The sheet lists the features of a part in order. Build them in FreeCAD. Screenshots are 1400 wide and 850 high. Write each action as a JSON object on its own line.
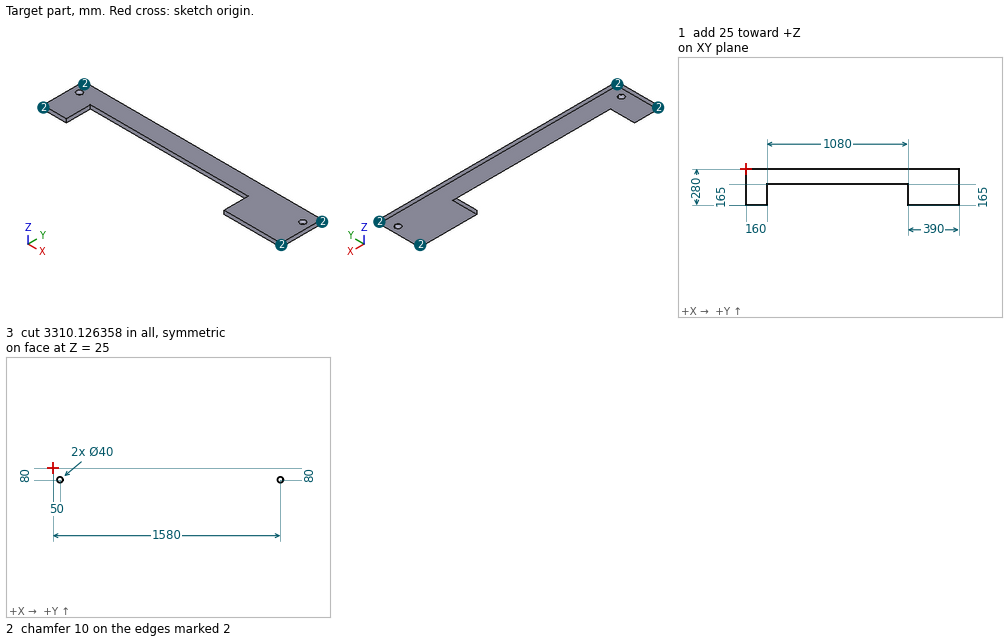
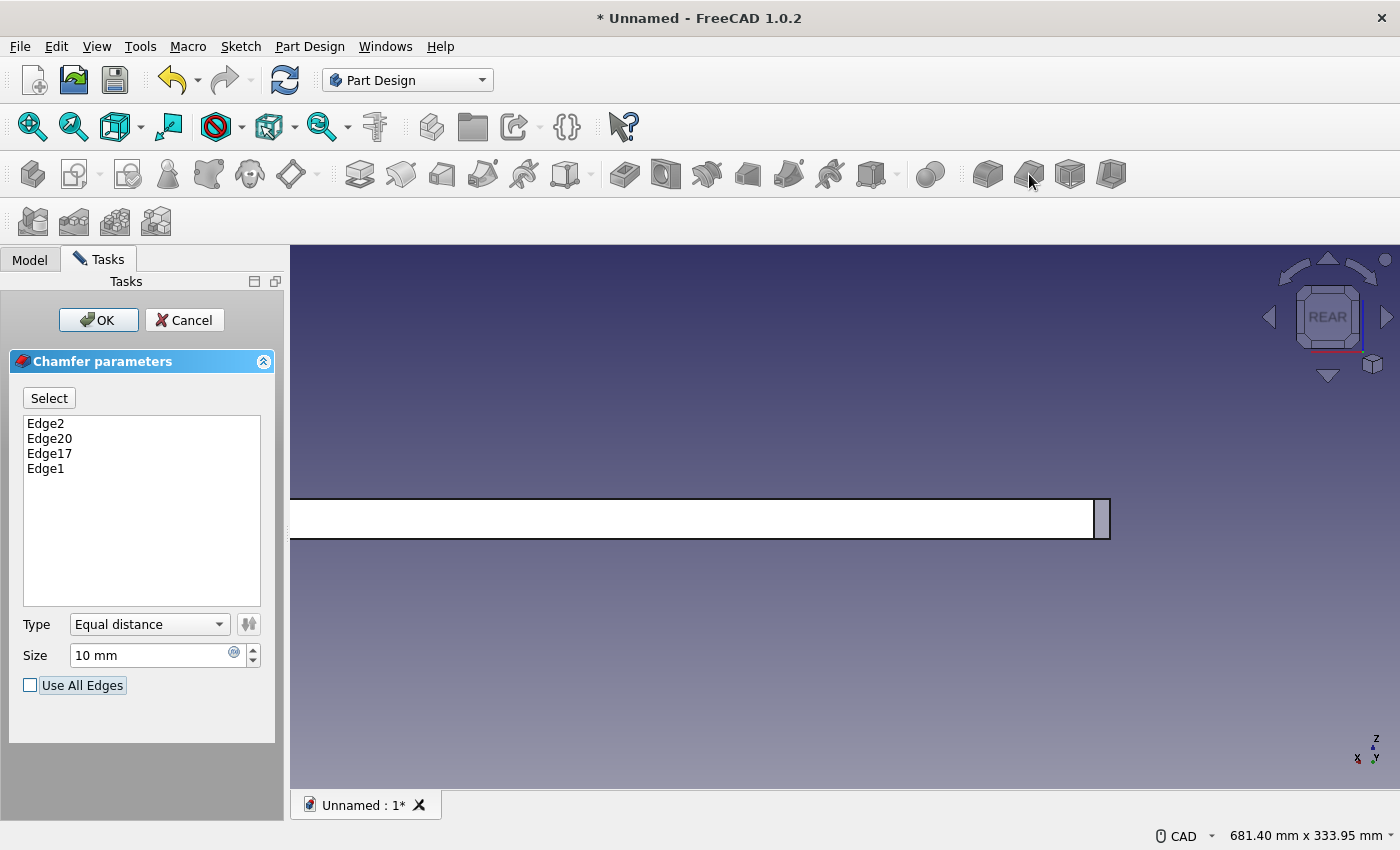
{"action": "left_click", "coordinate": [99, 320]}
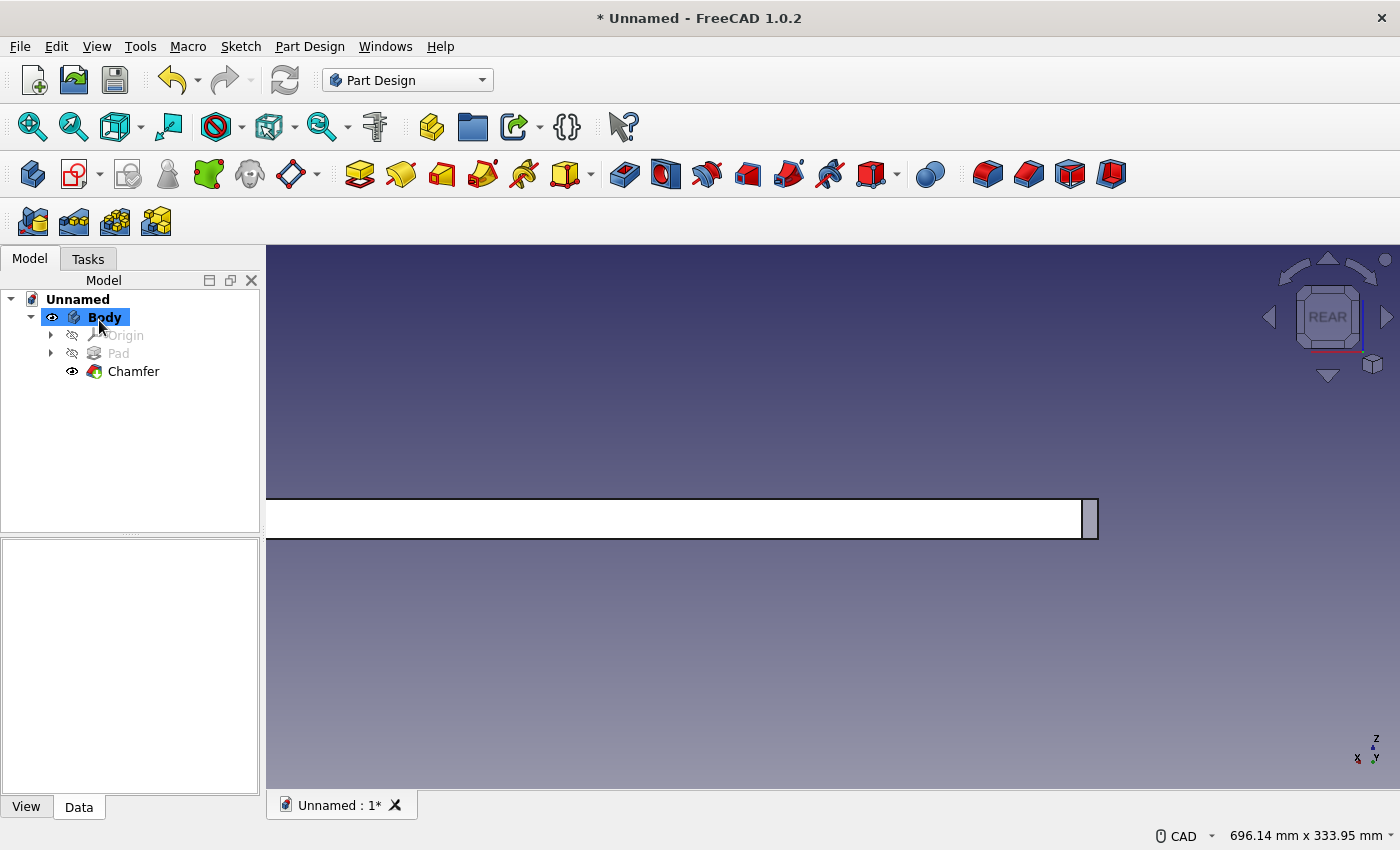
{"action": "key", "text": "v f"}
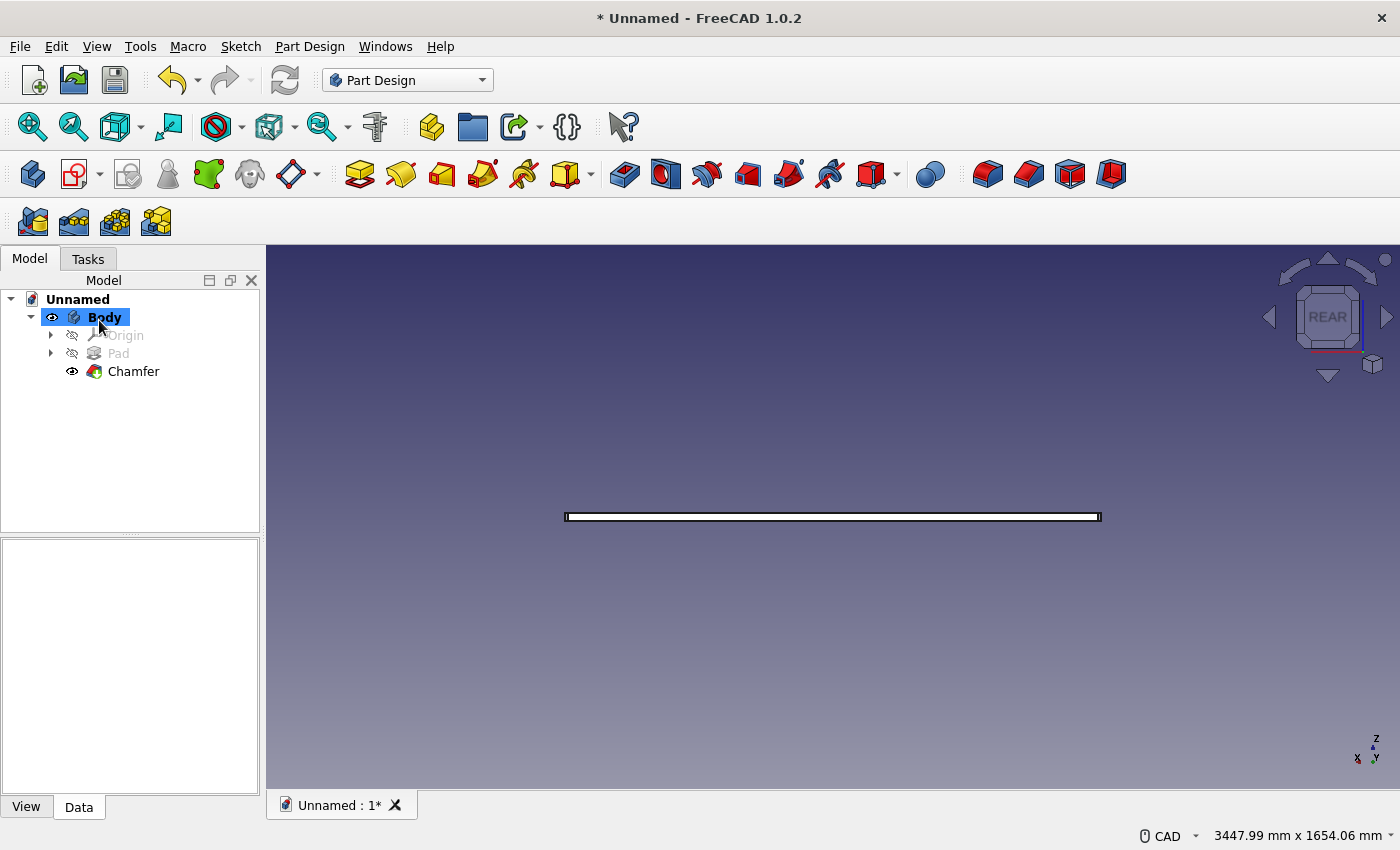
{"action": "key", "text": "0"}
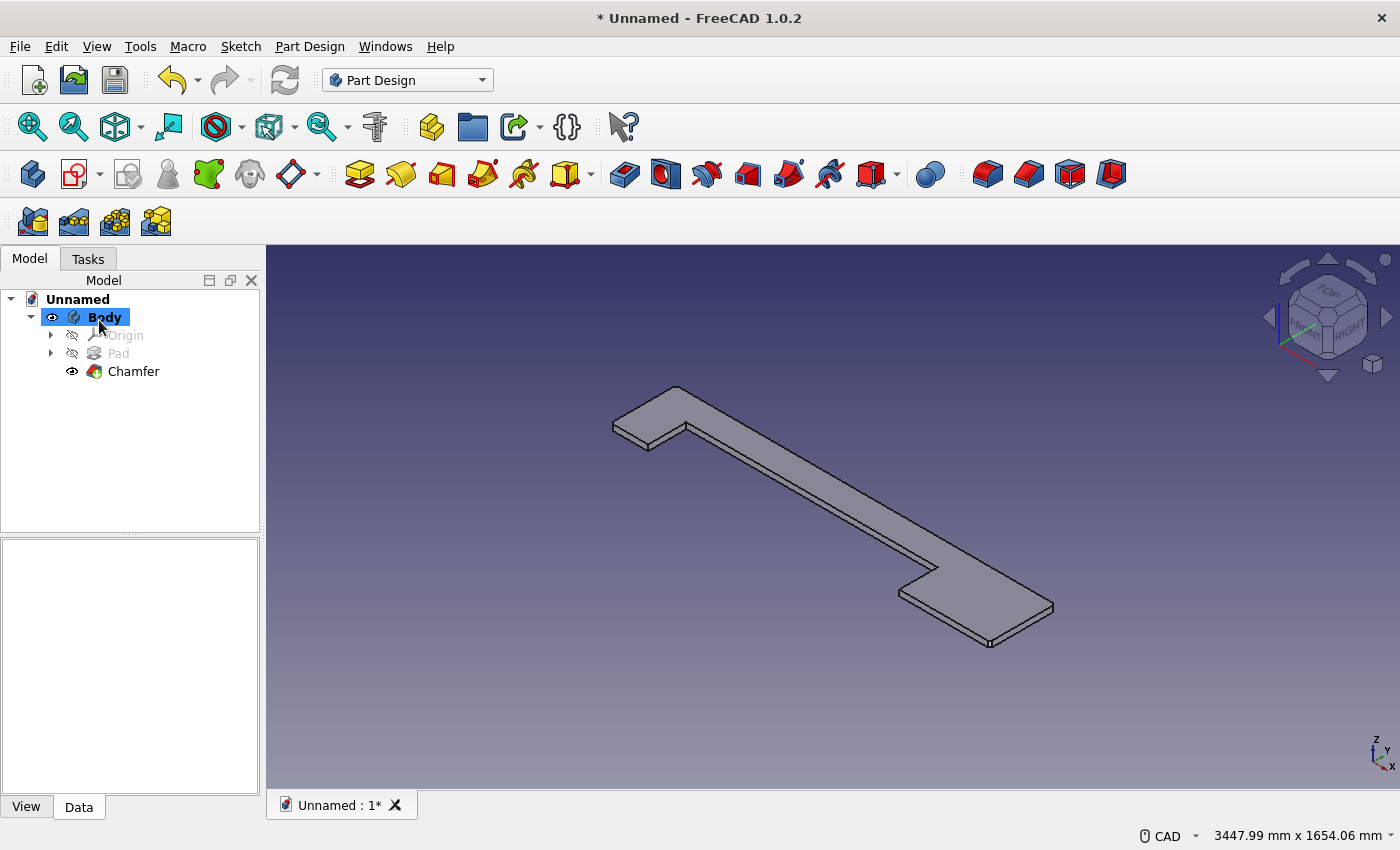
{"action": "left_click", "coordinate": [995, 606]}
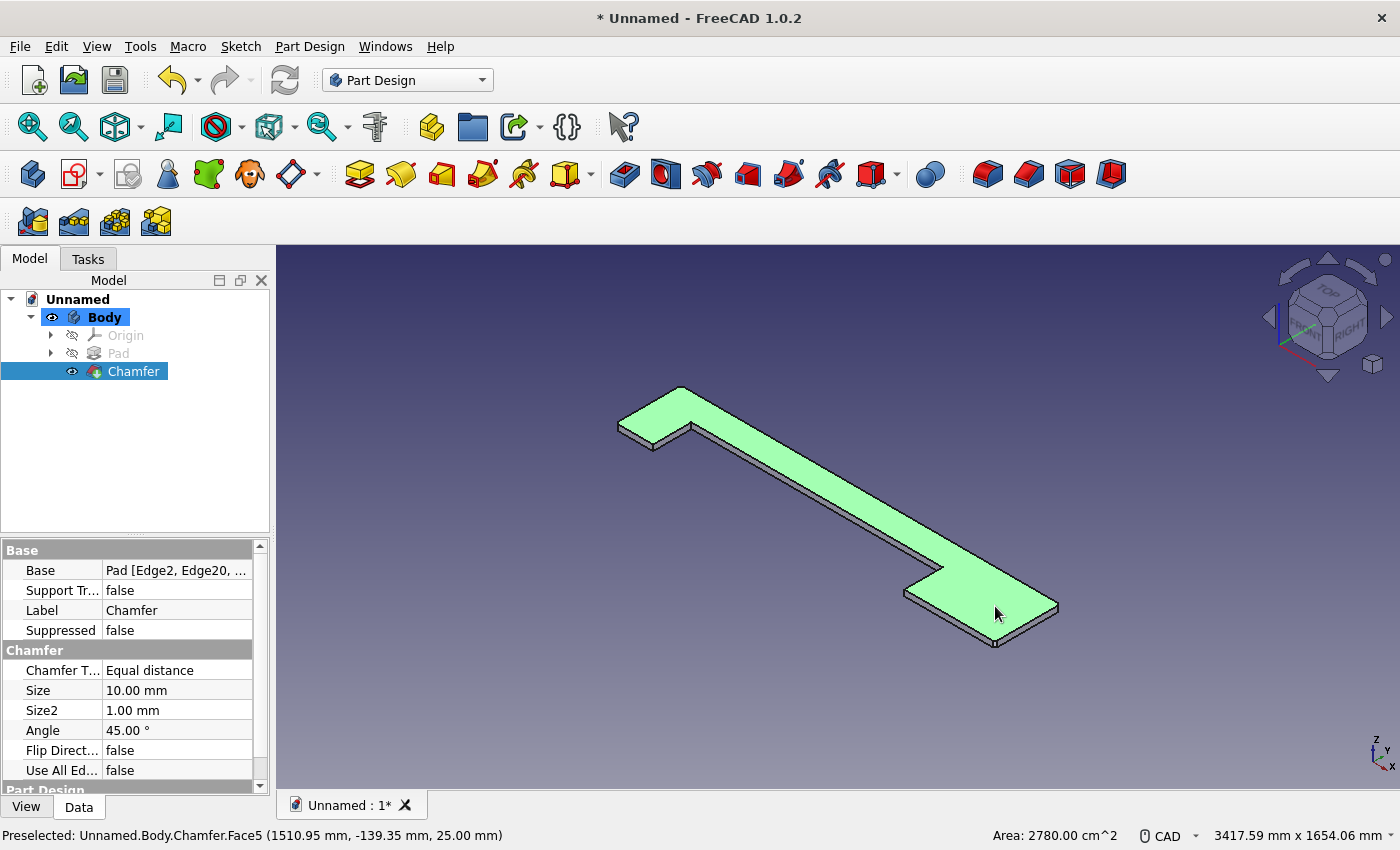
{"action": "left_click", "coordinate": [74, 174]}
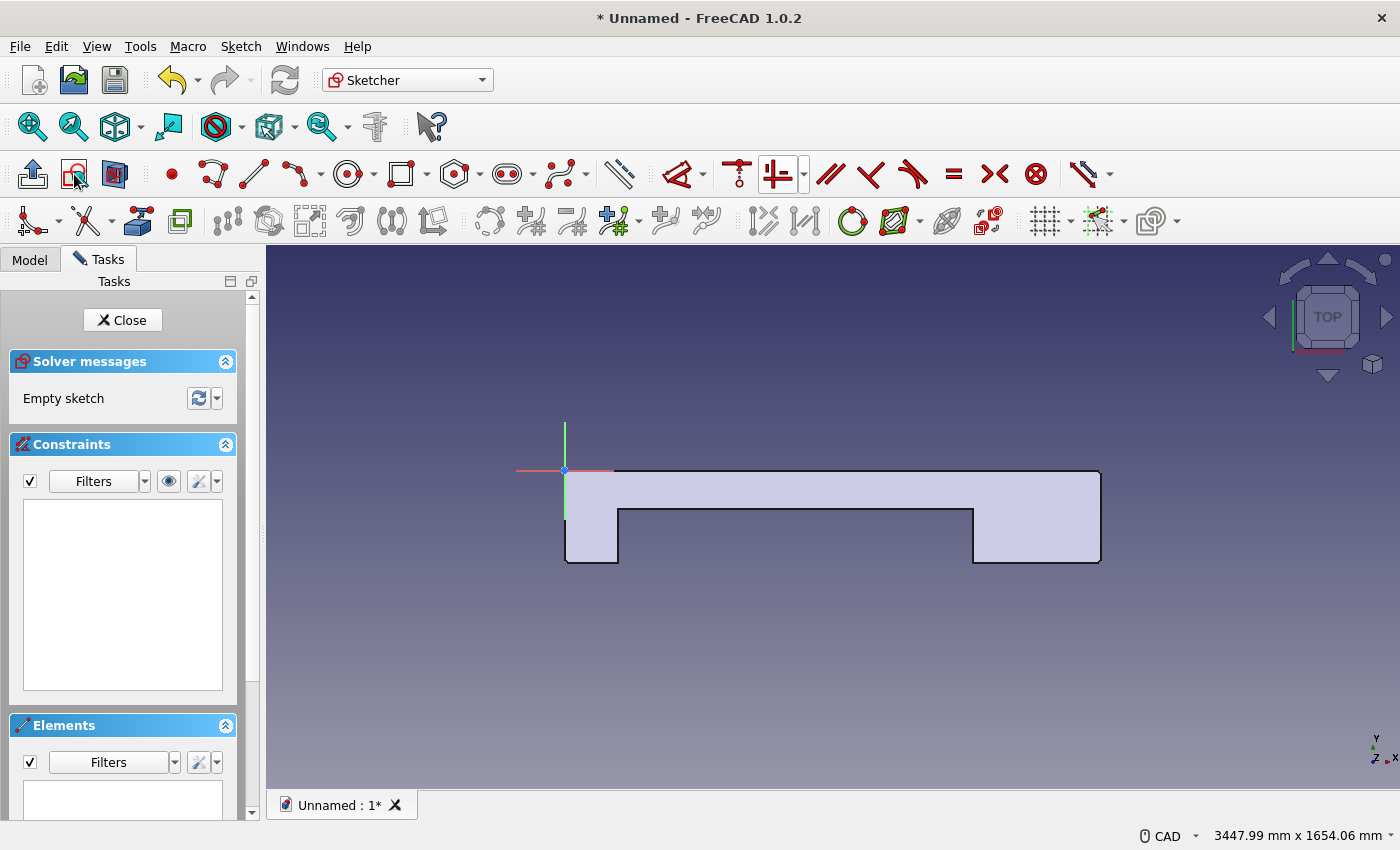
{"action": "key", "text": "g c"}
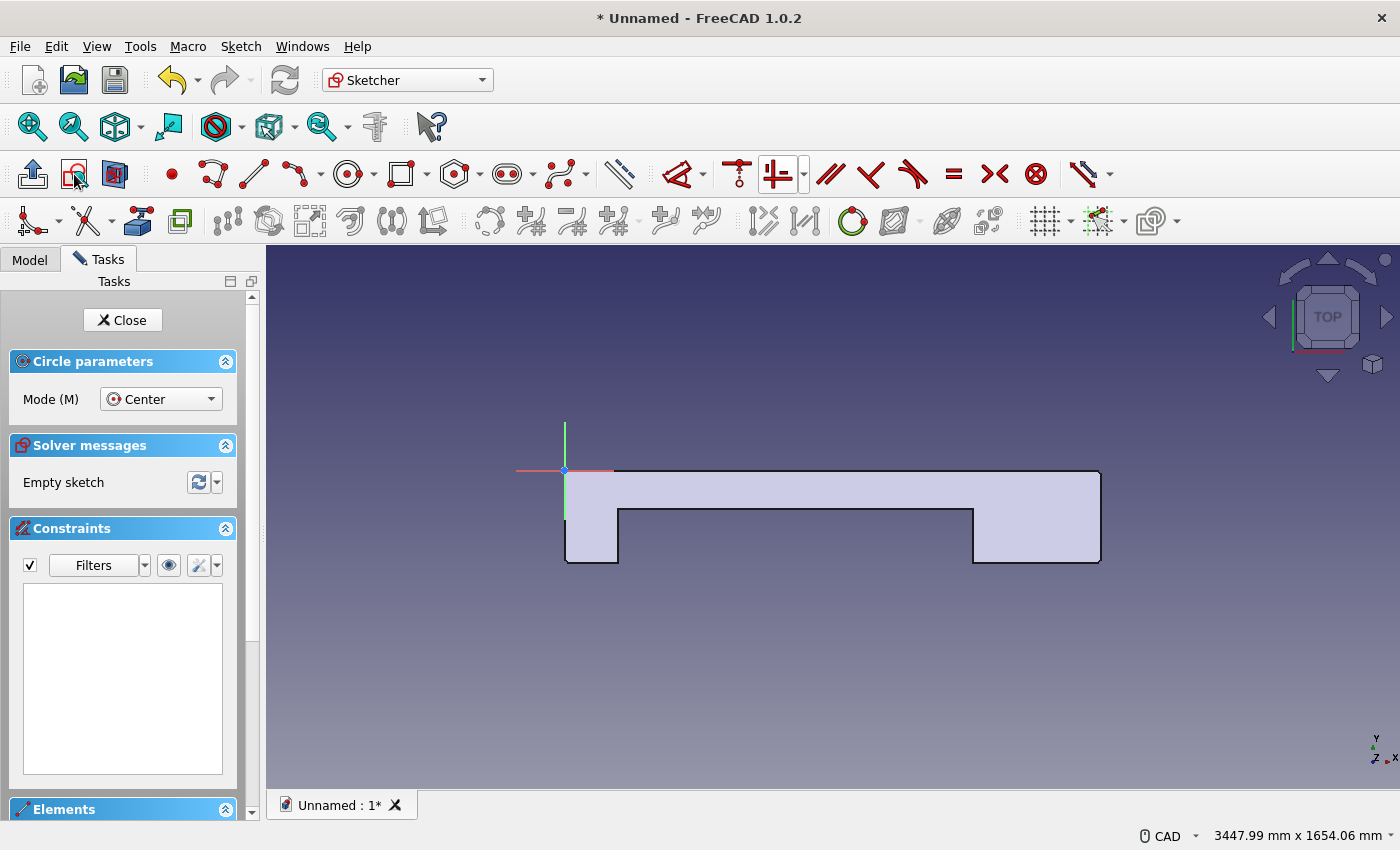
{"action": "scroll", "coordinate": [581, 497], "scroll_direction": "up", "scroll_amount": 7}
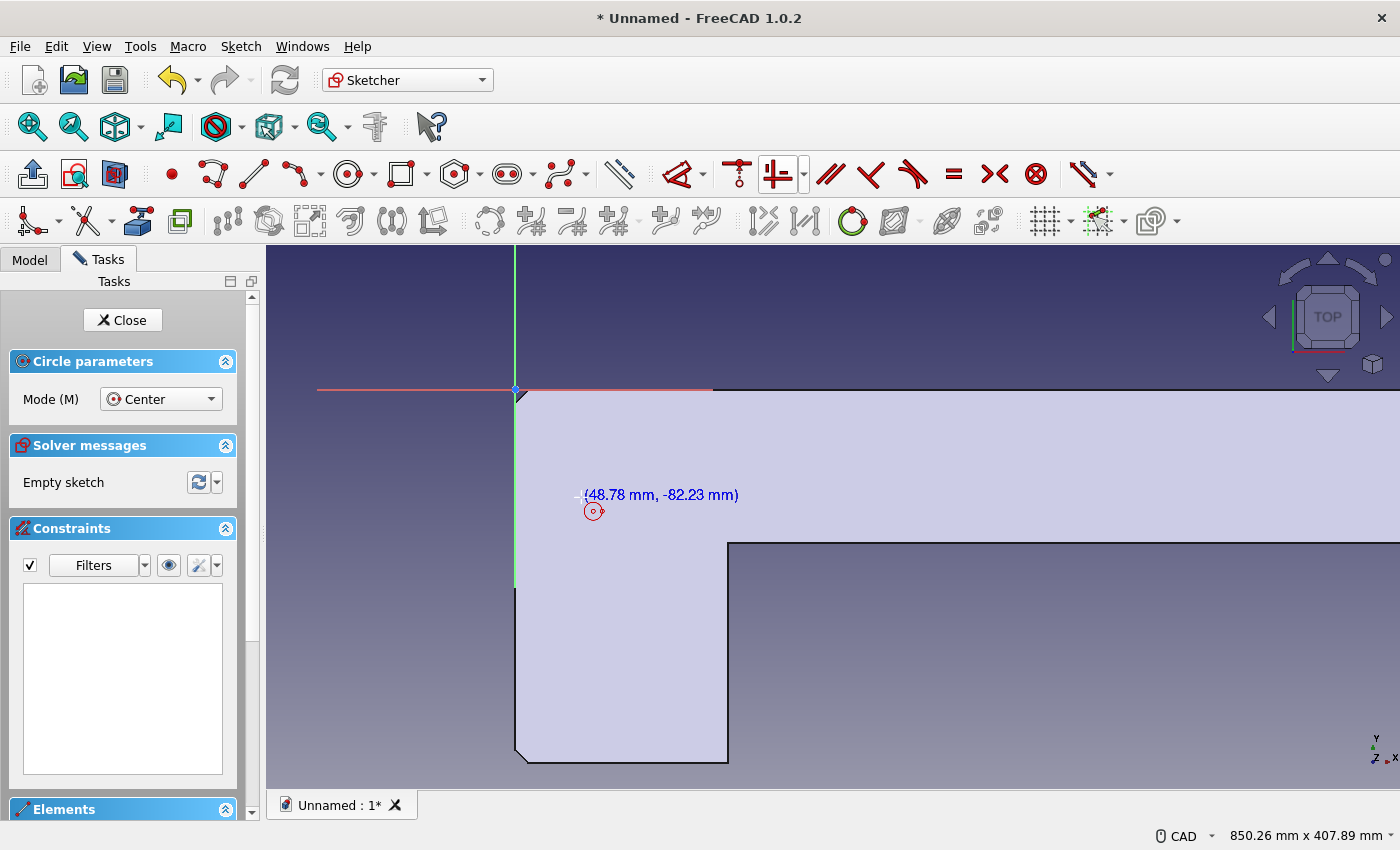
{"action": "scroll", "coordinate": [412, 543], "scroll_direction": "down", "scroll_amount": 6}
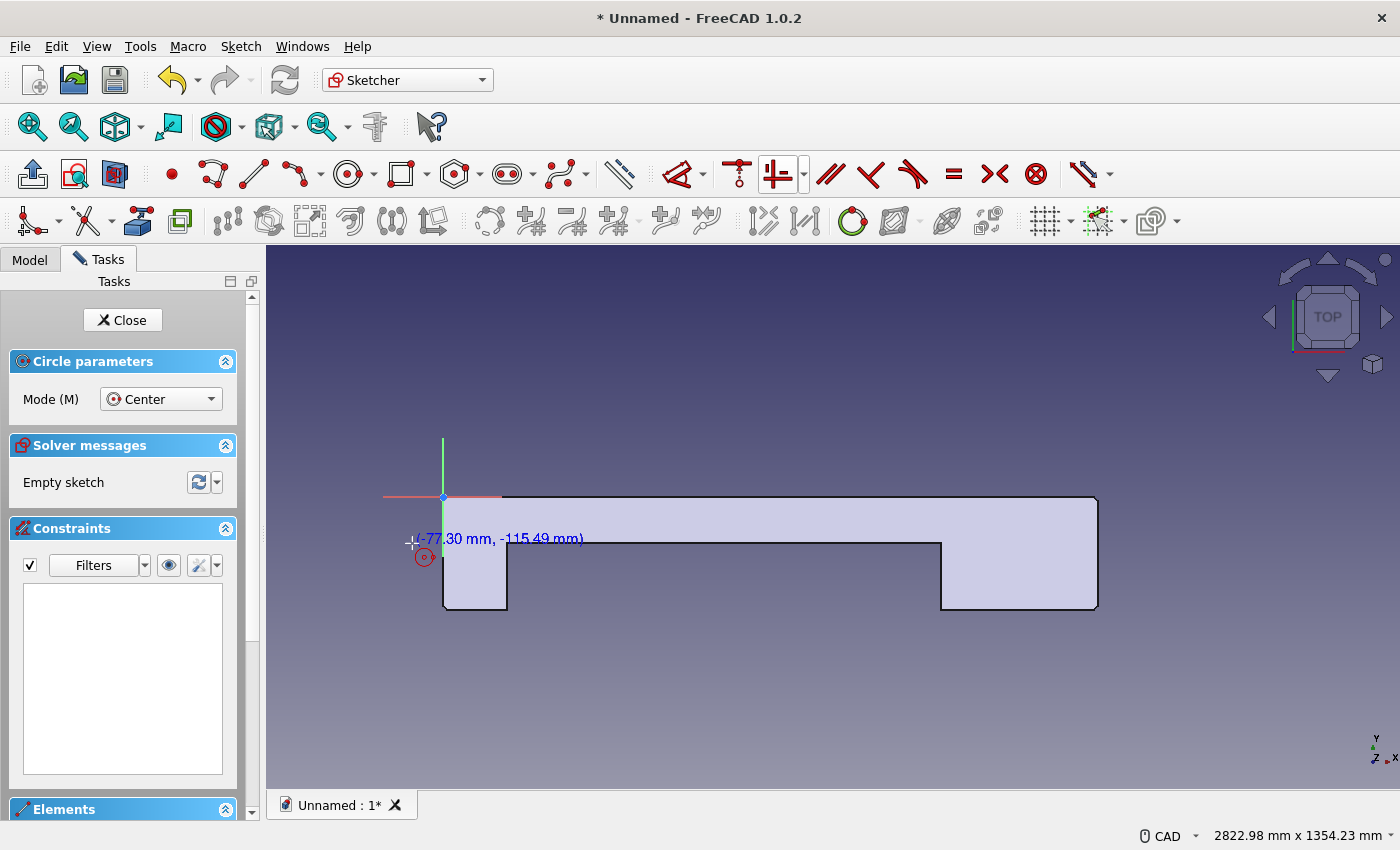
{"action": "left_click", "coordinate": [463, 529]}
{"action": "mouse_move", "coordinate": [469, 524]}